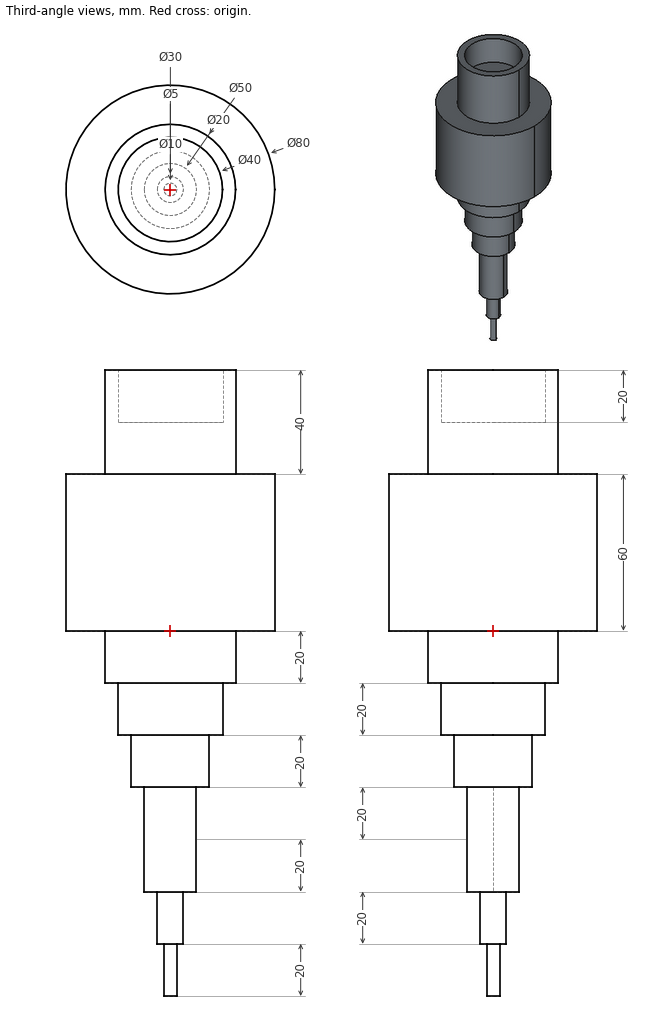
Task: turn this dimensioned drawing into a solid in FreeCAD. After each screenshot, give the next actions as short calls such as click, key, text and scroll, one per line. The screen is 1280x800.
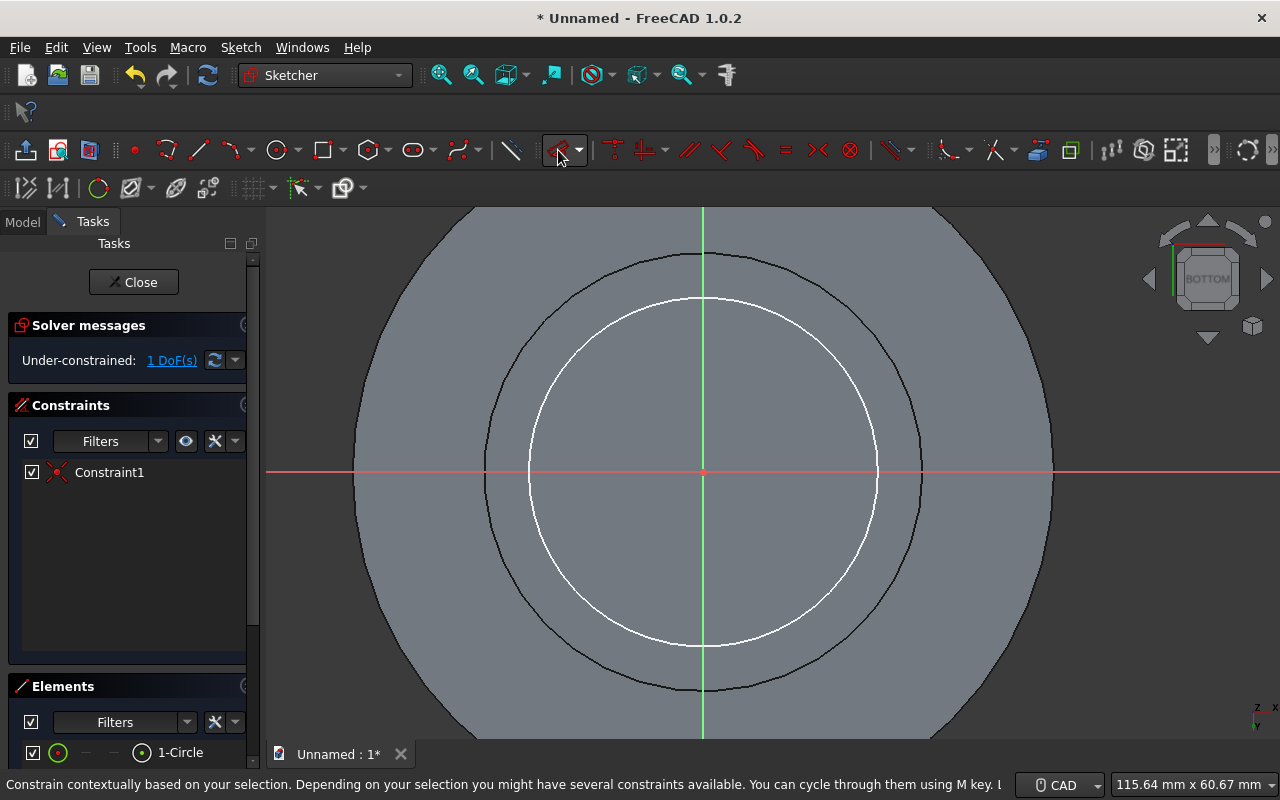
click(826, 348)
click(848, 325)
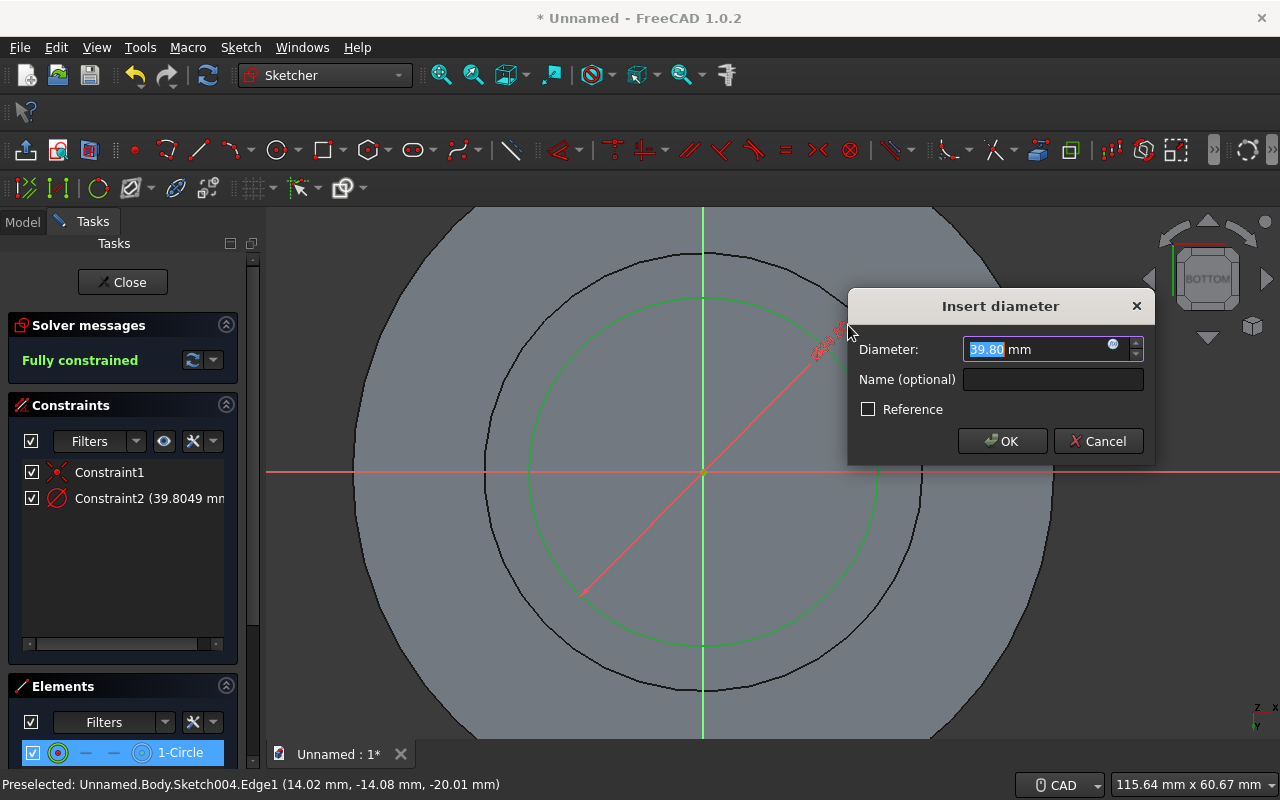
text(40)
key(Return)
key(Escape)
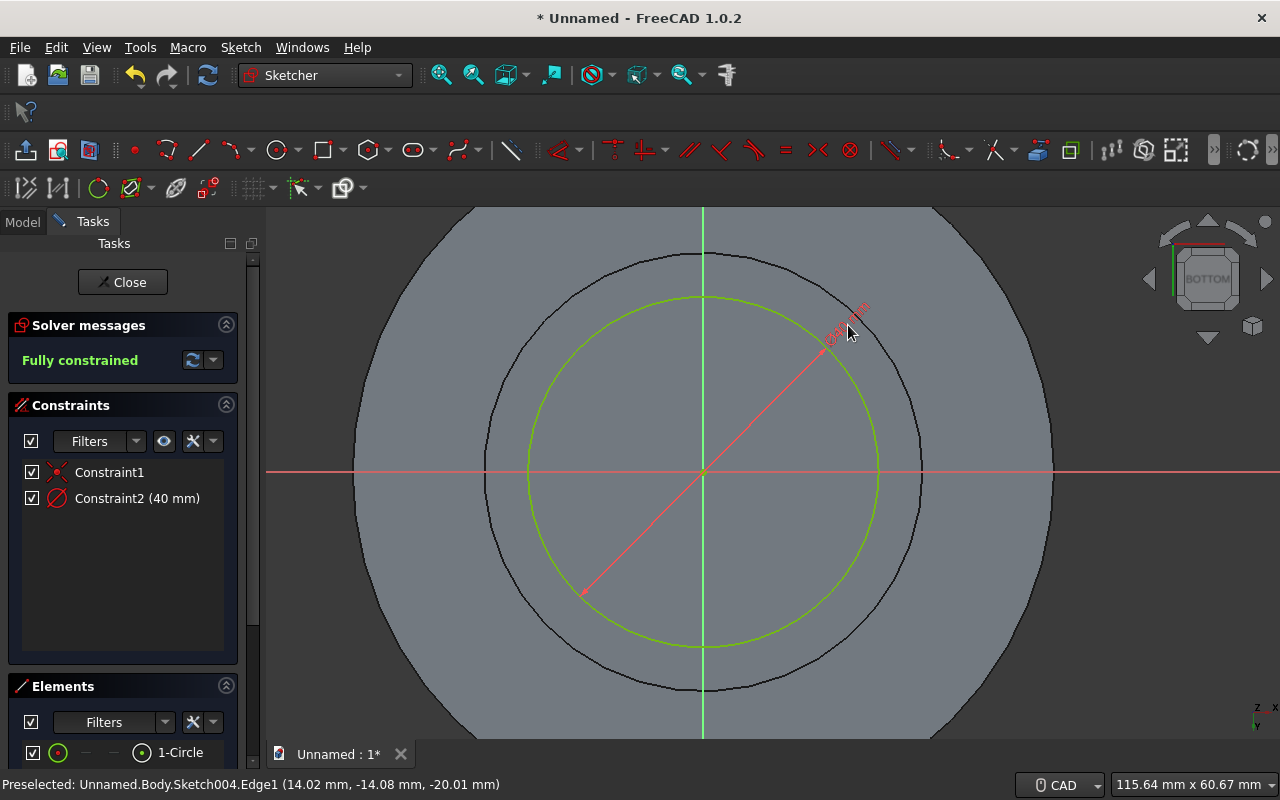
click(123, 282)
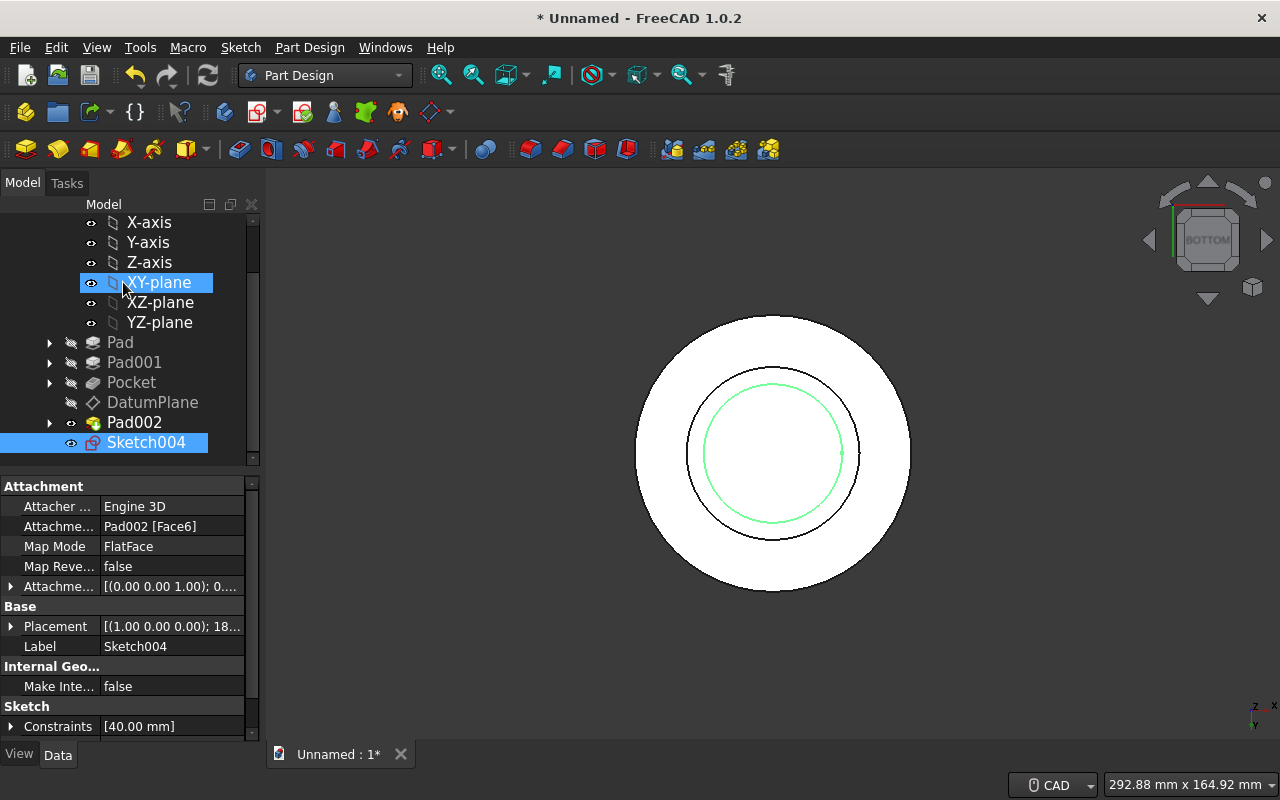
click(26, 150)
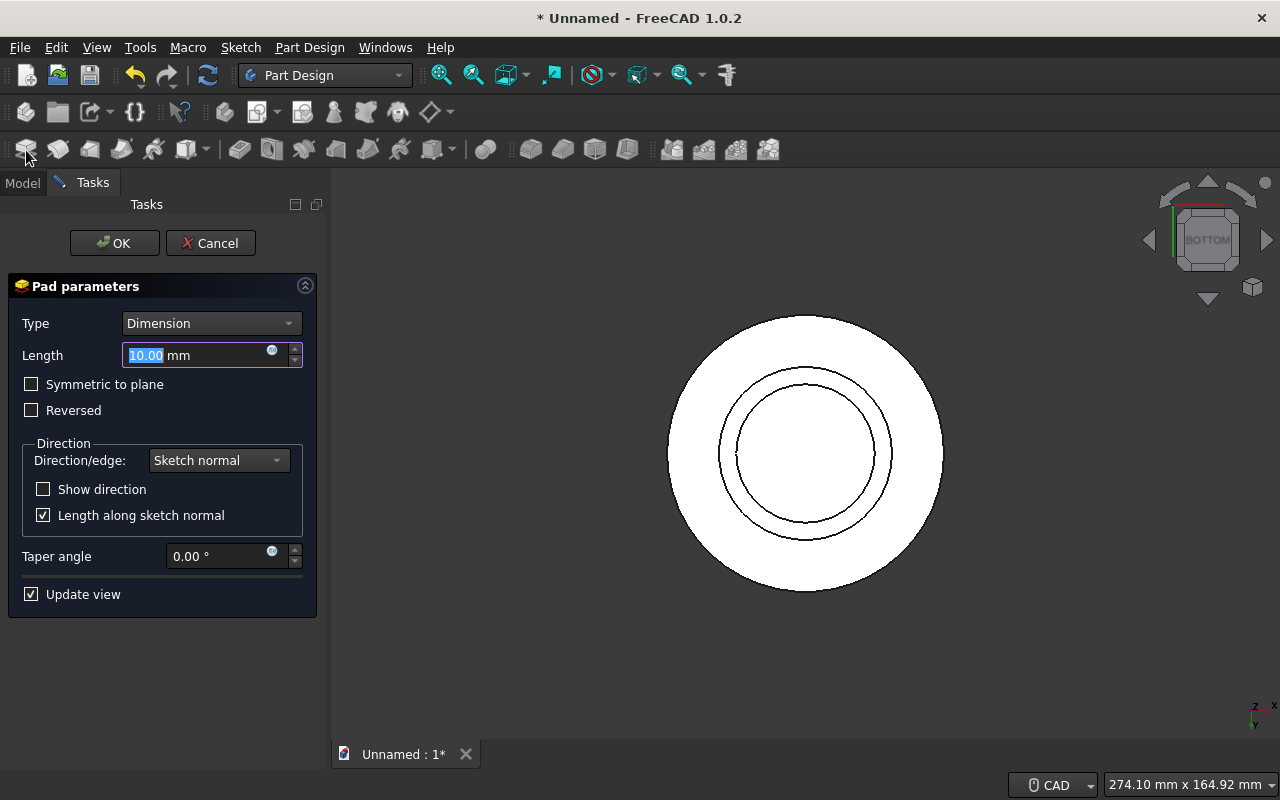
text(20)
key(Tab)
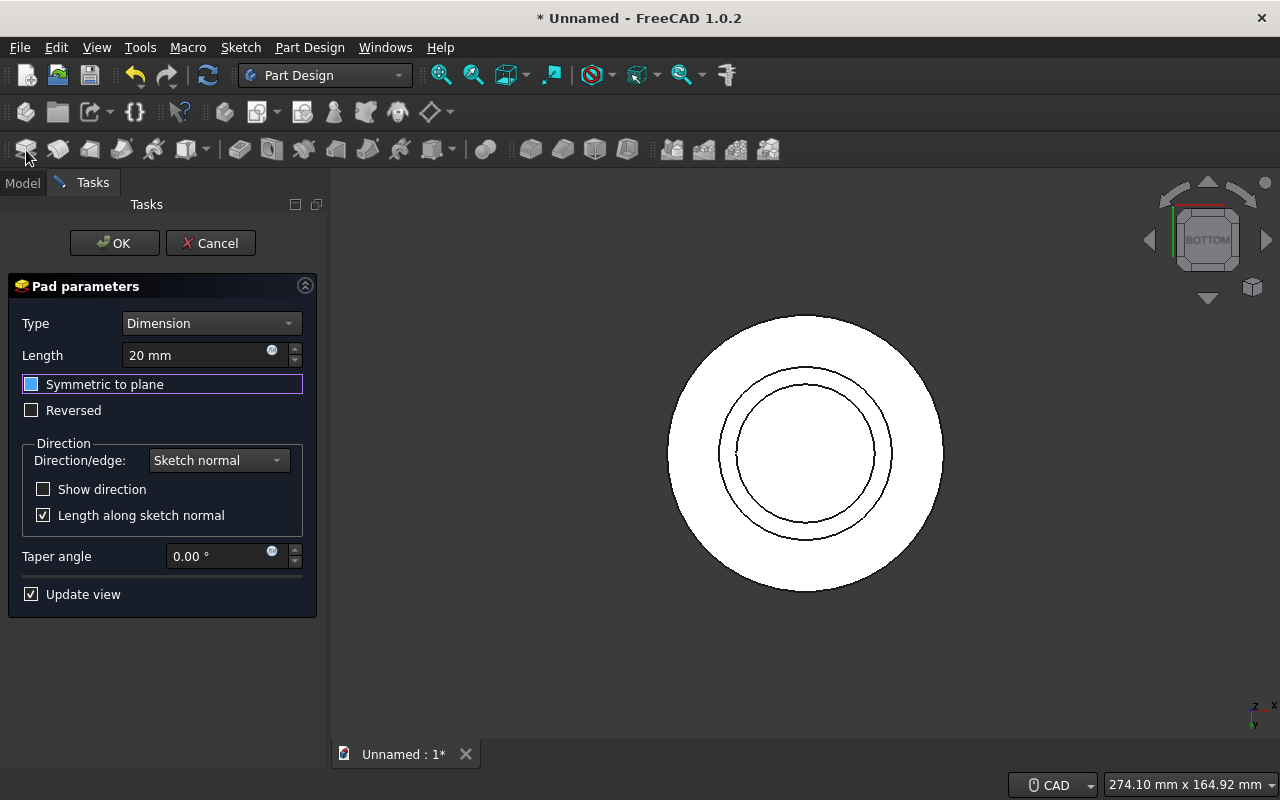
click(115, 243)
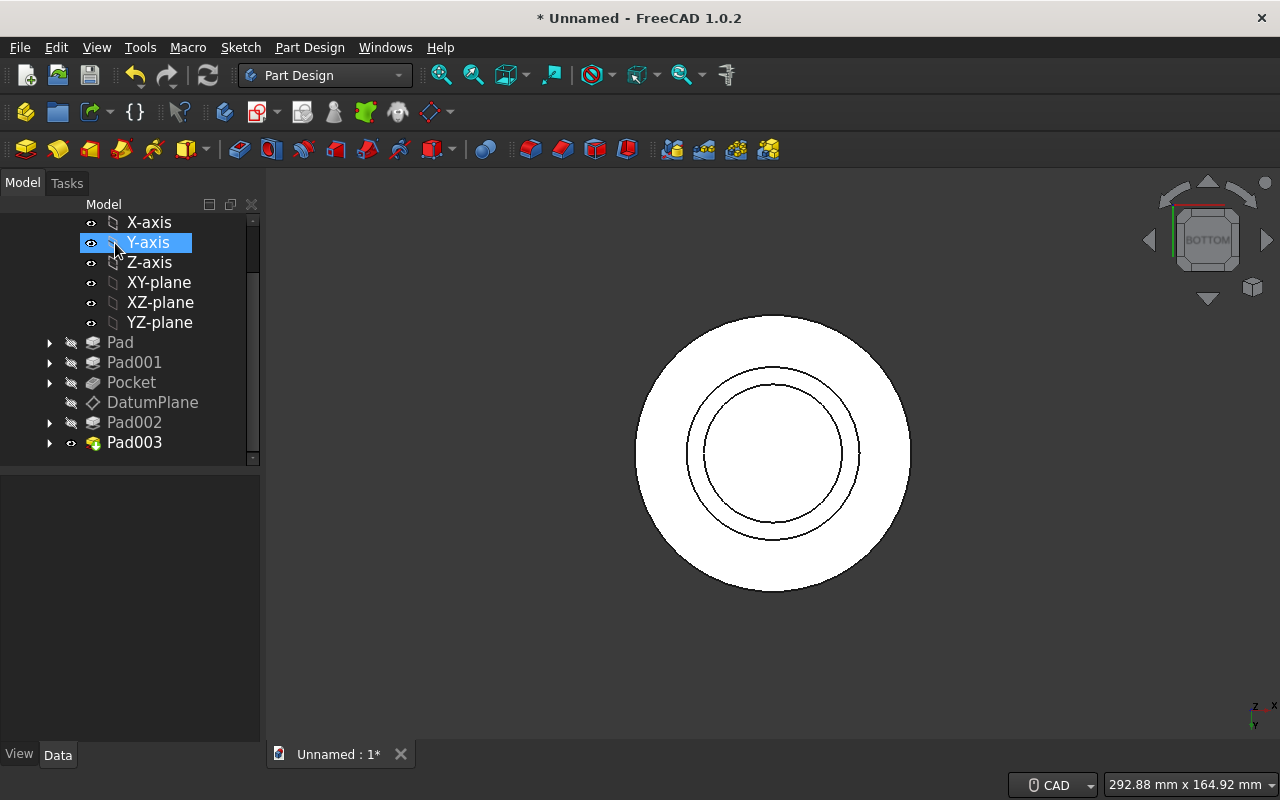
click(773, 452)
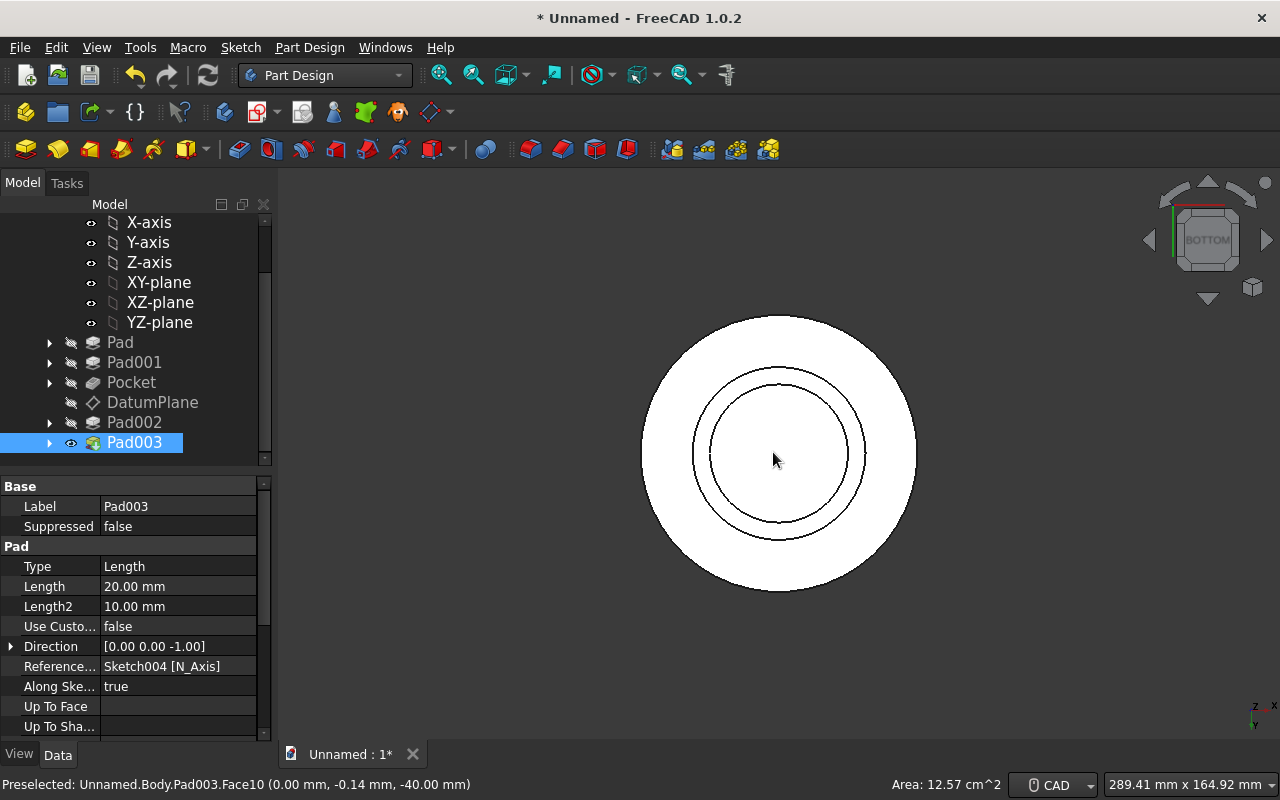
click(258, 112)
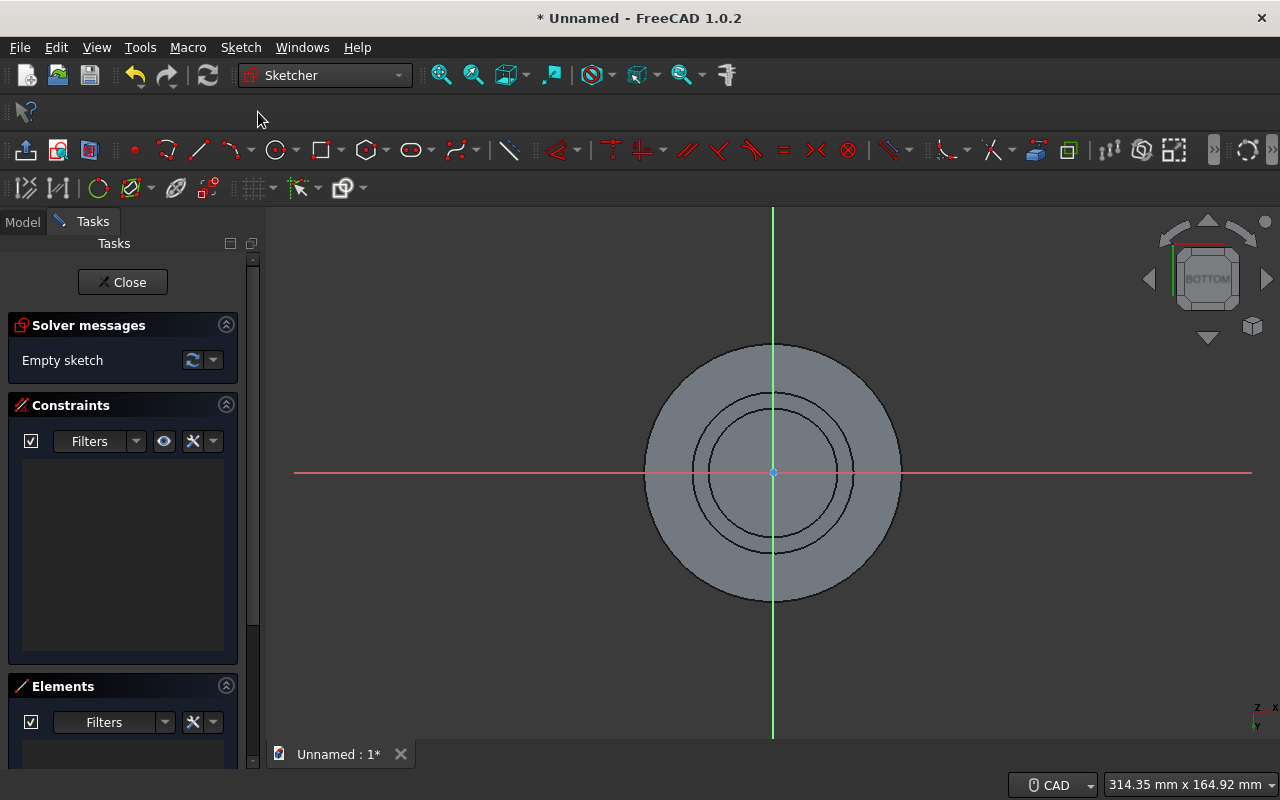
scroll(803, 473, up, 6)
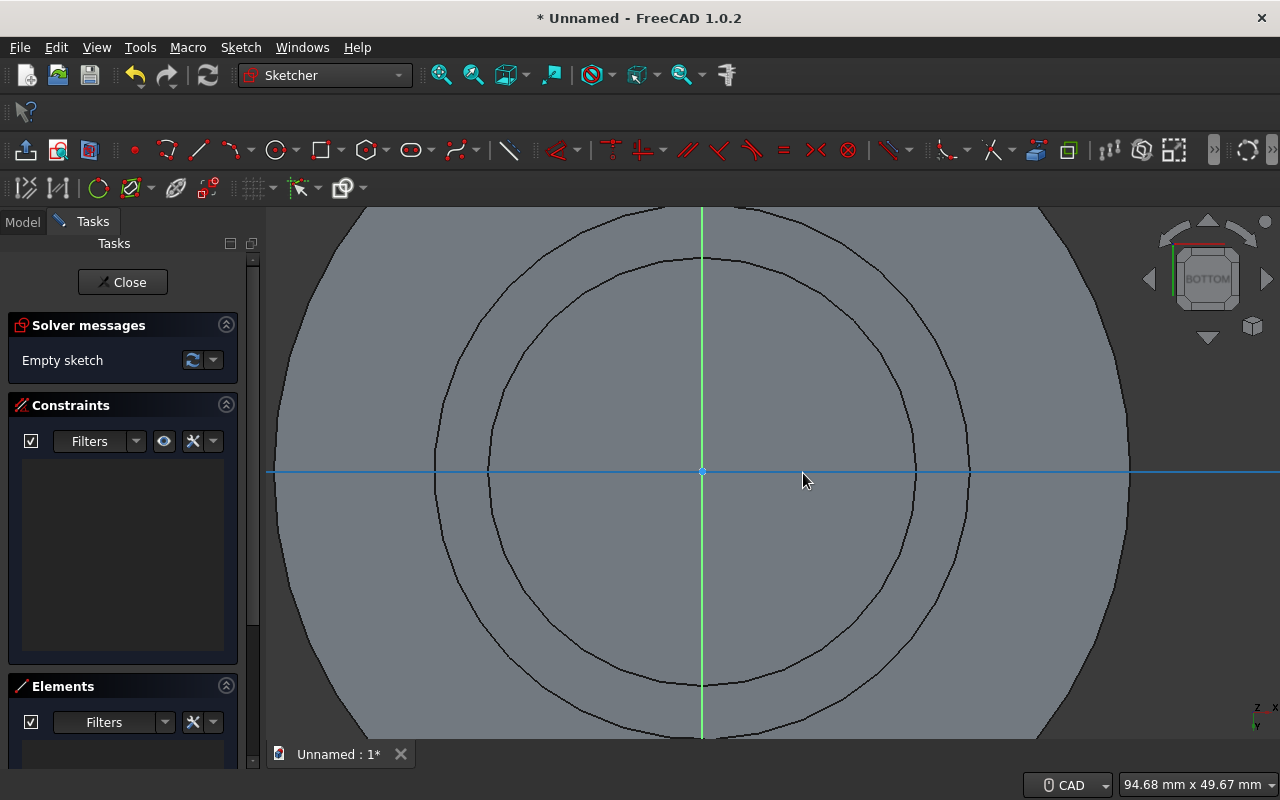
click(276, 150)